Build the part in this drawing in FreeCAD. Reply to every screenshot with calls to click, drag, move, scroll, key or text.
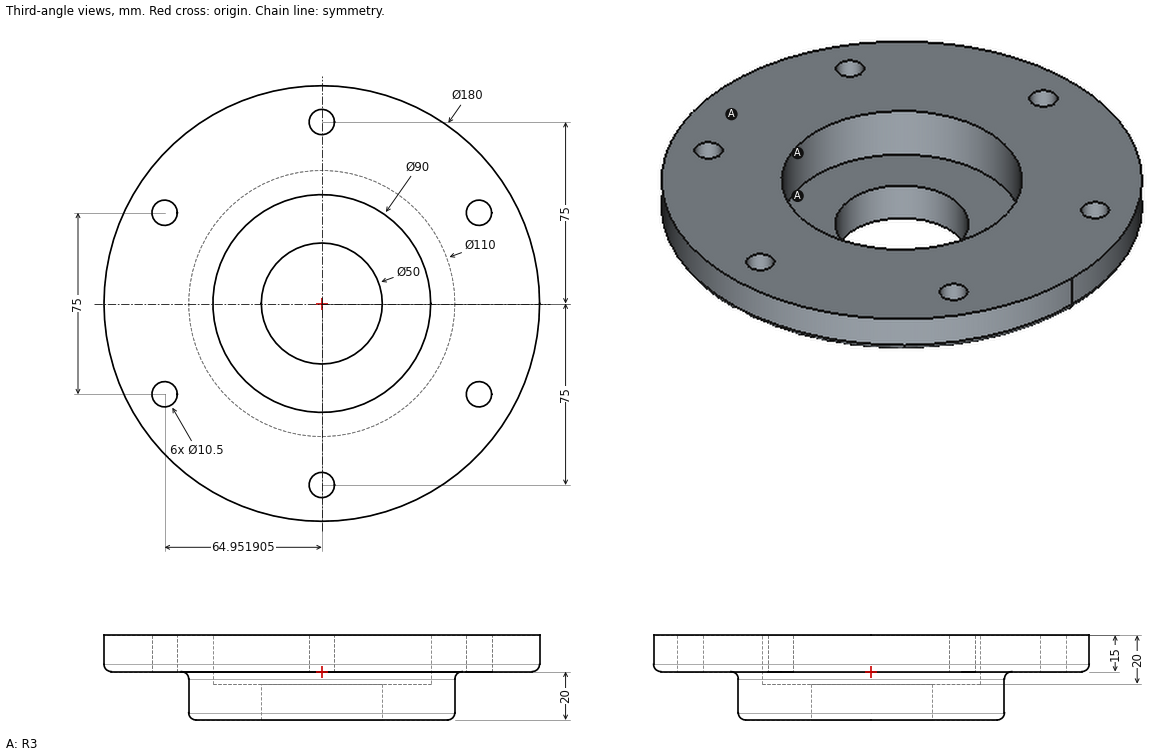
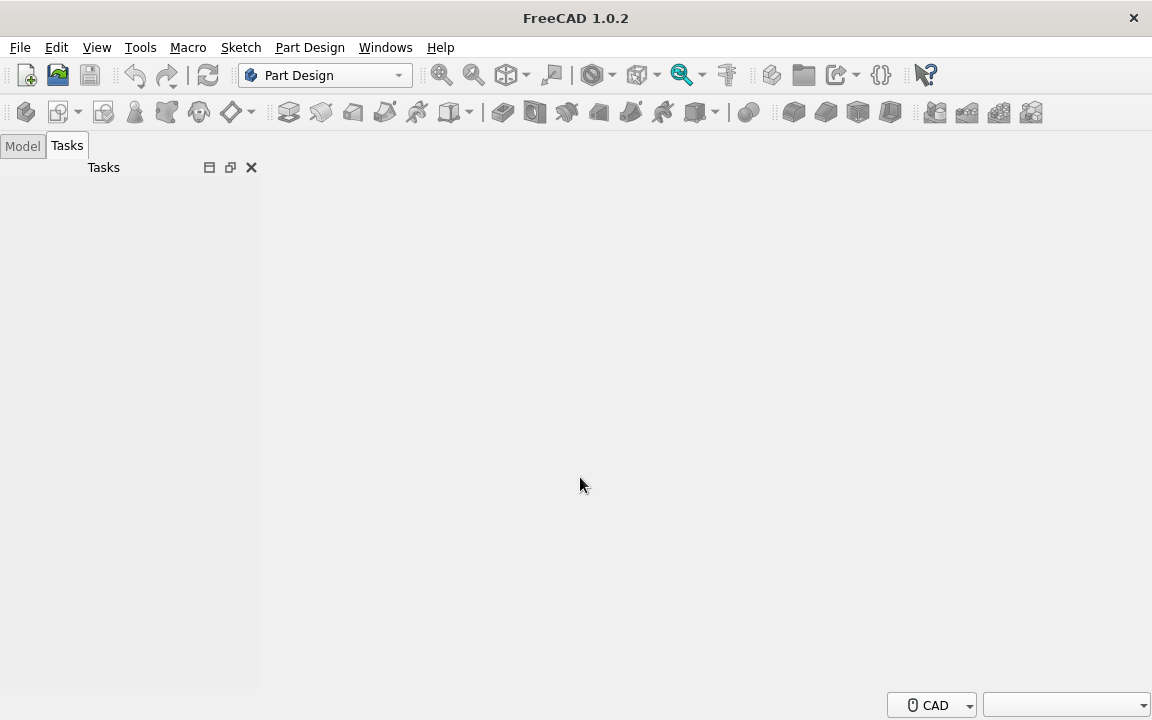
key(ctrl+n)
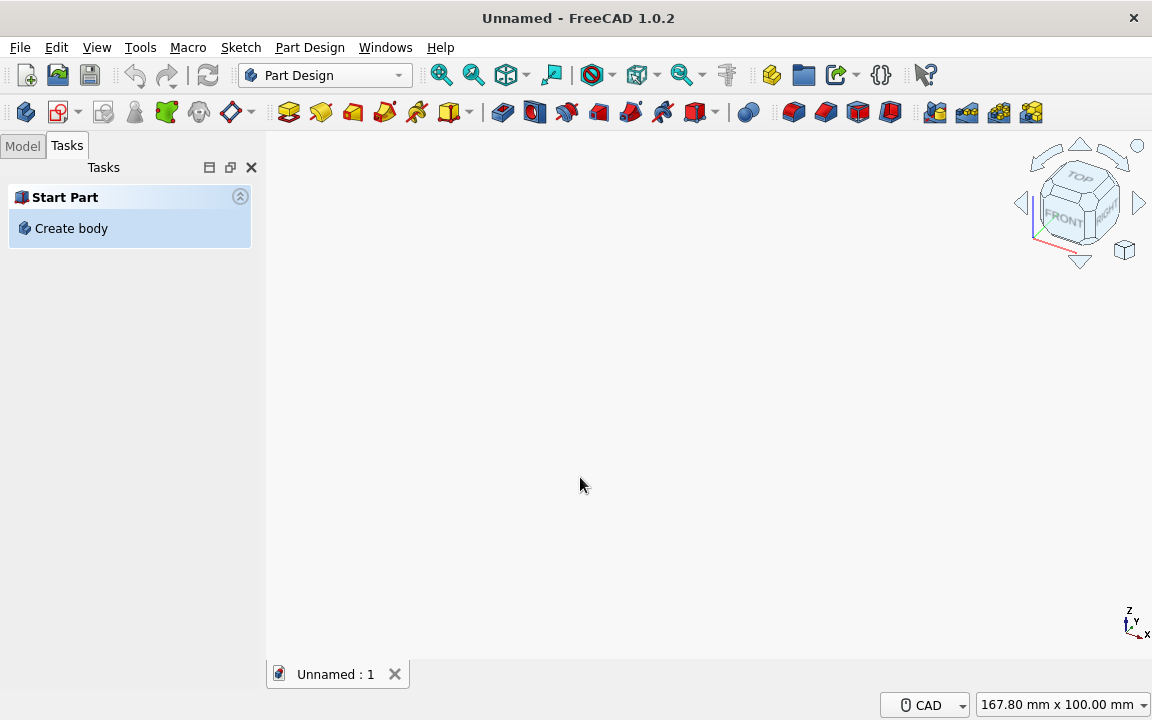
click(58, 112)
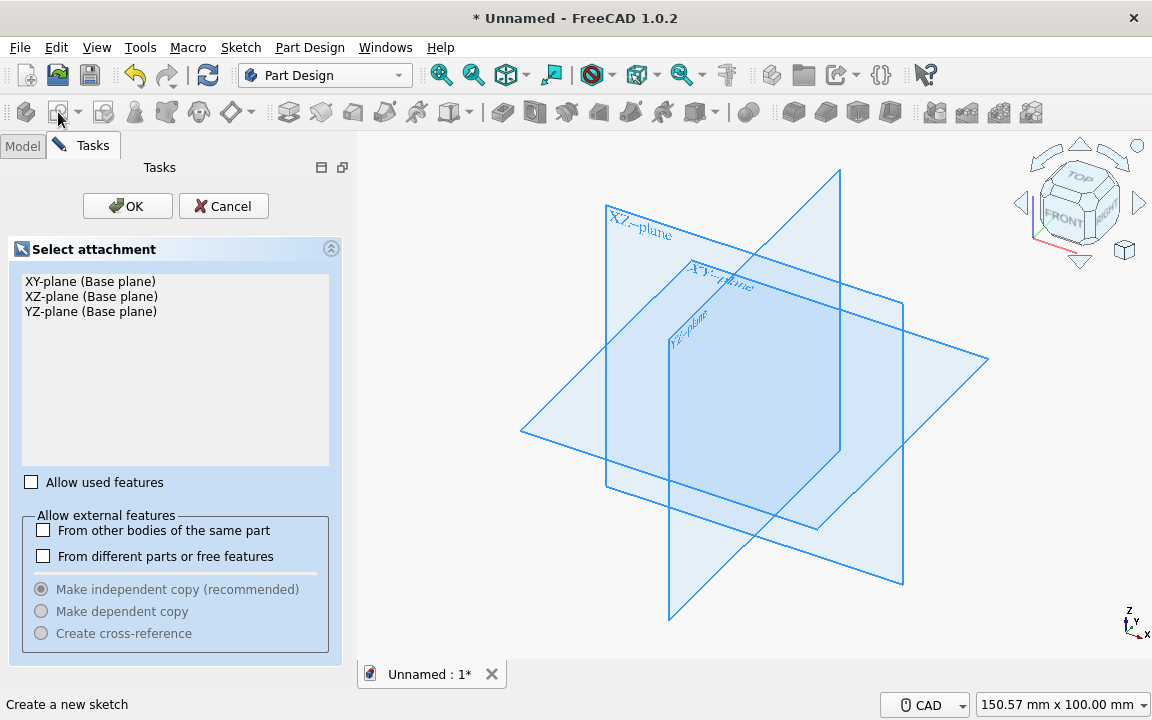
click(82, 282)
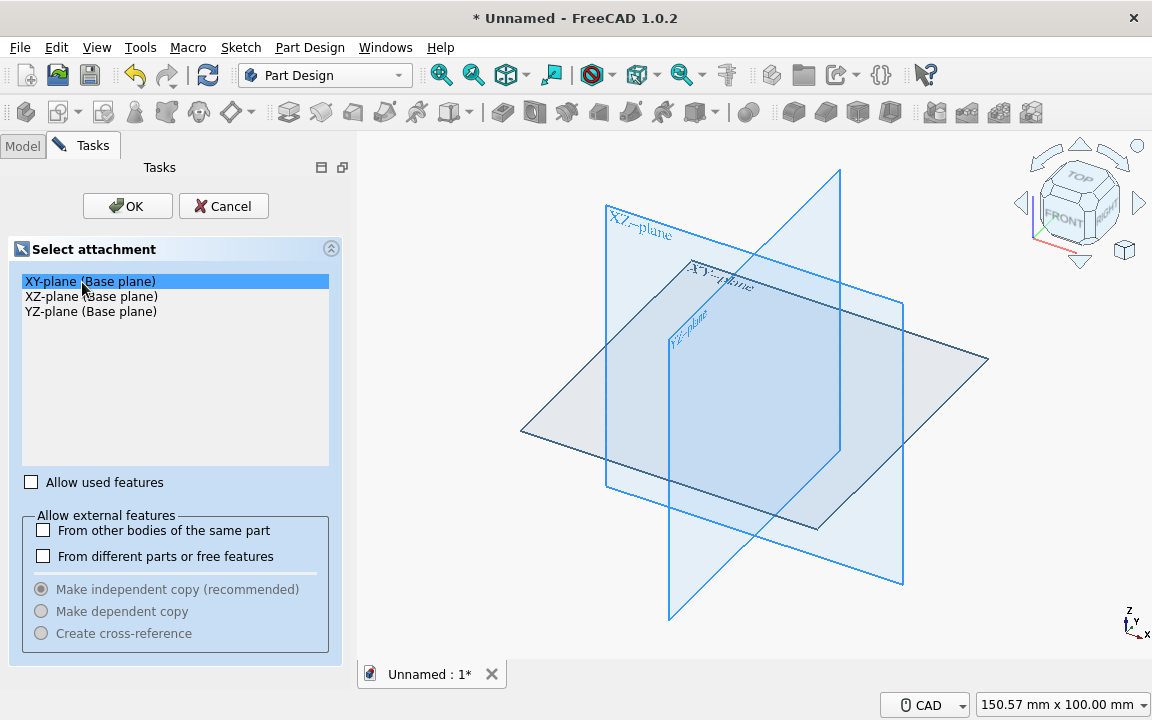
click(128, 206)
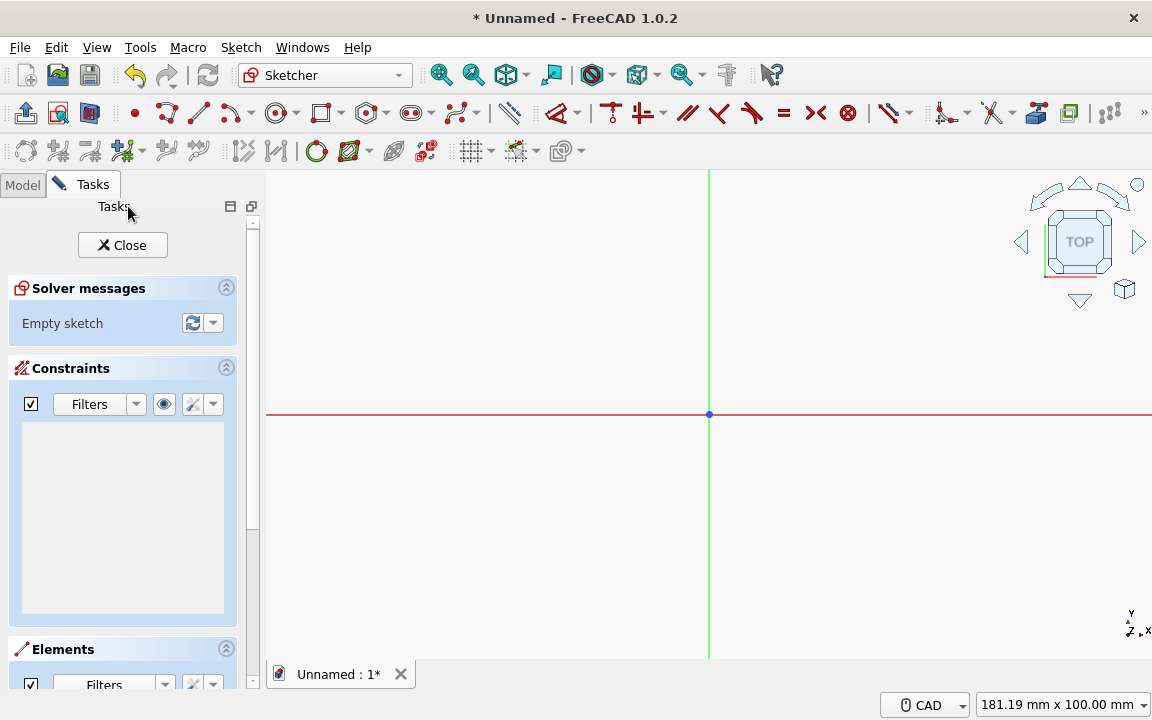
scroll(601, 414, down, 5)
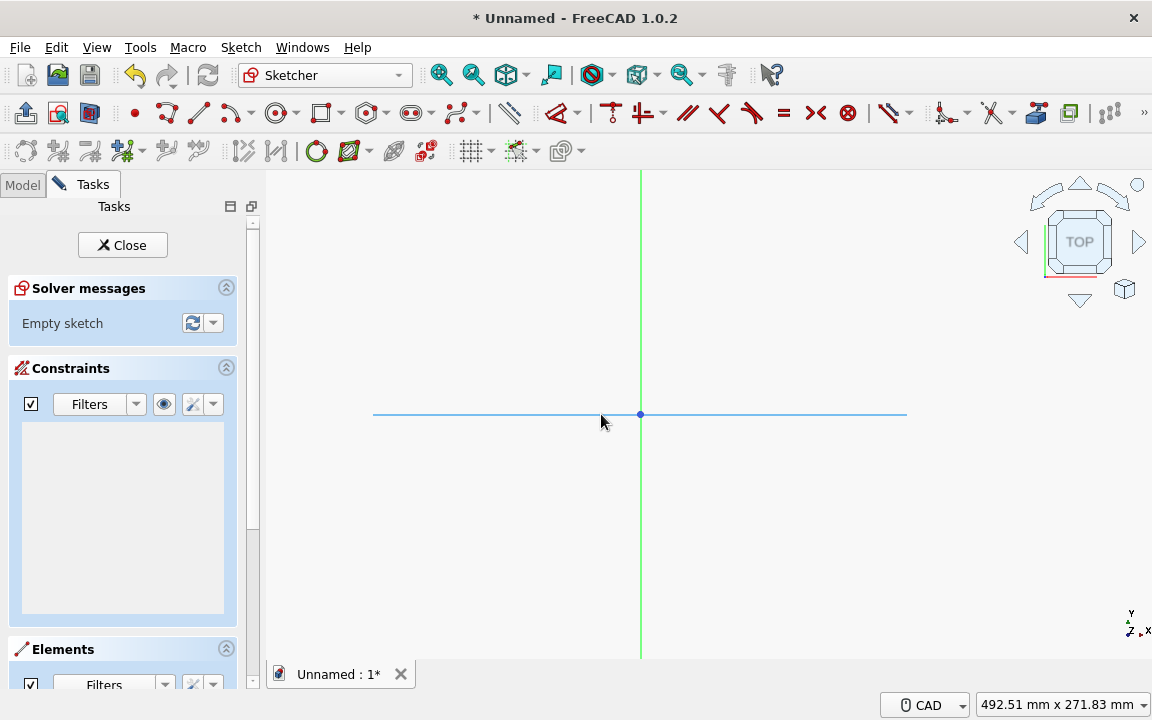
key(g)
key(c)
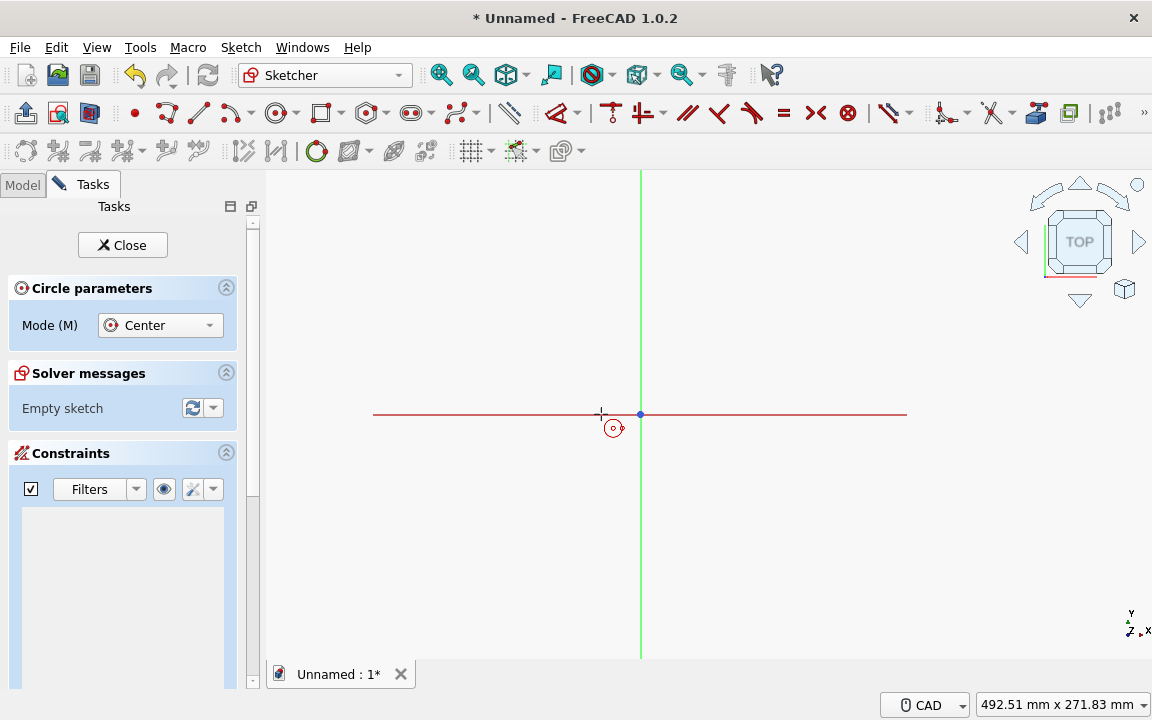
click(641, 414)
move(755, 300)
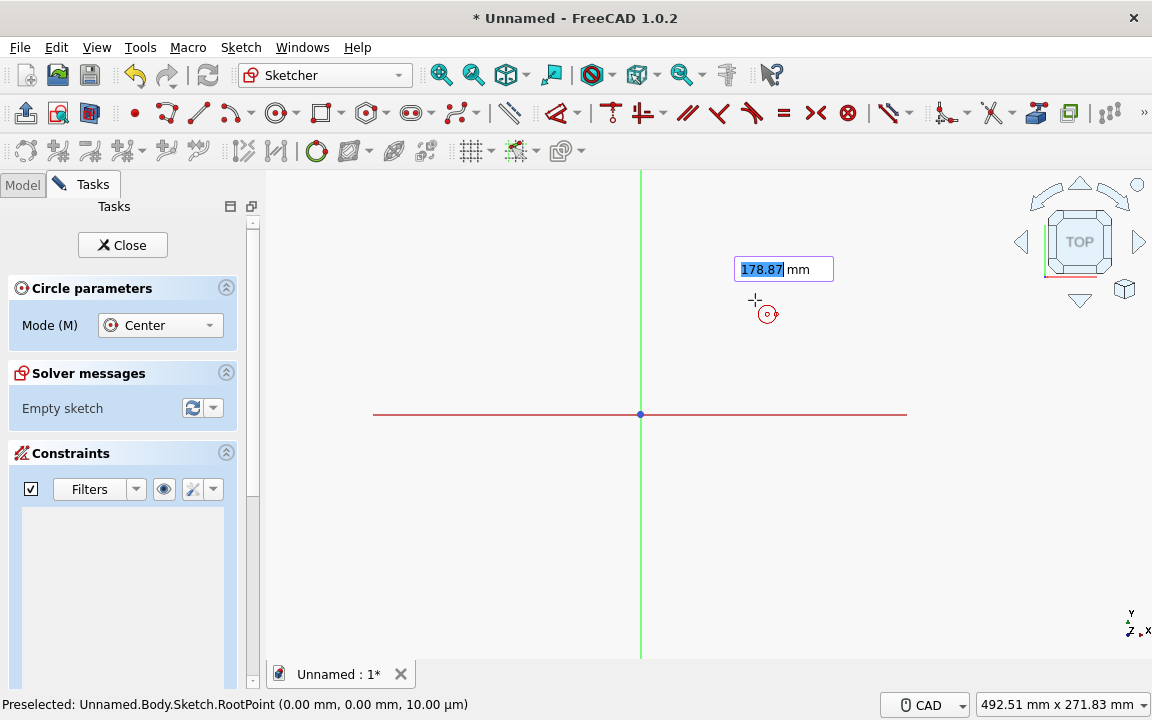
text(180)
key(Return)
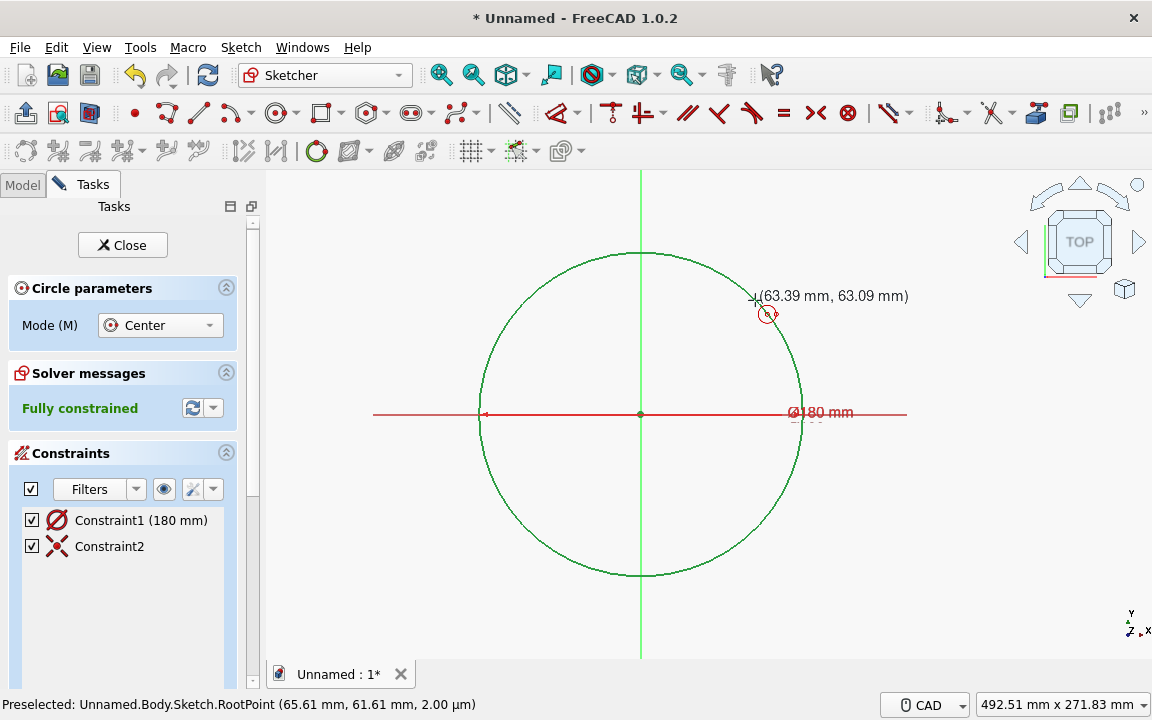
scroll(524, 482, up, 5)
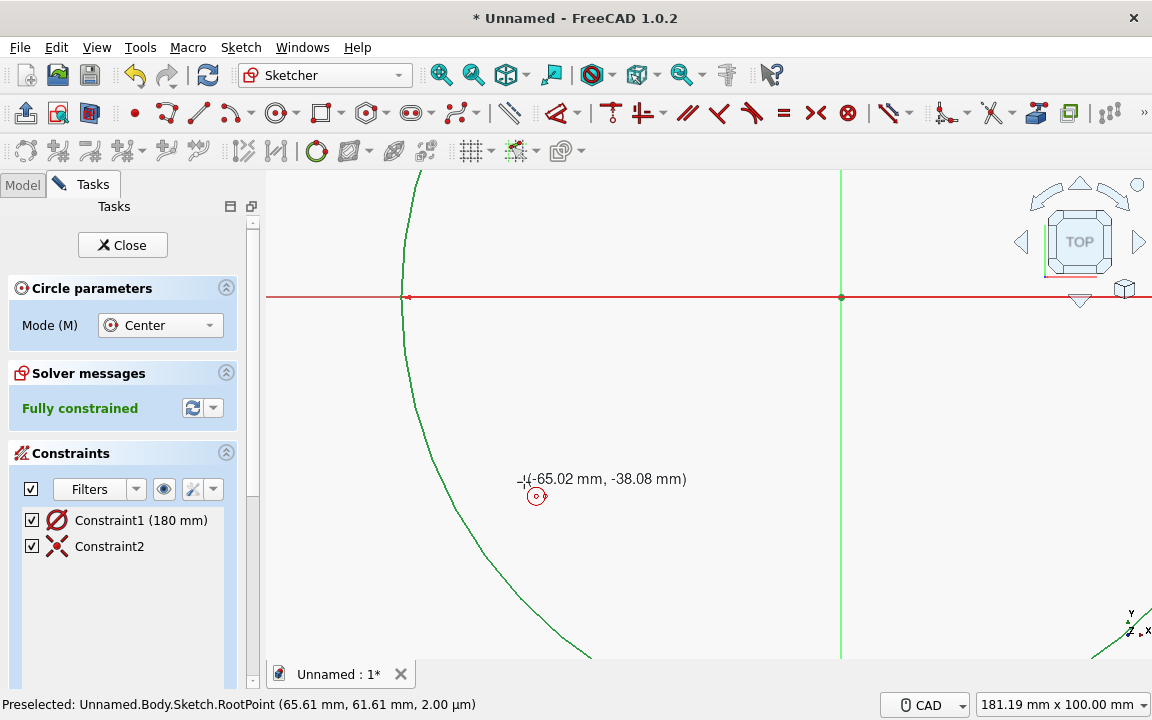
click(524, 481)
move(542, 463)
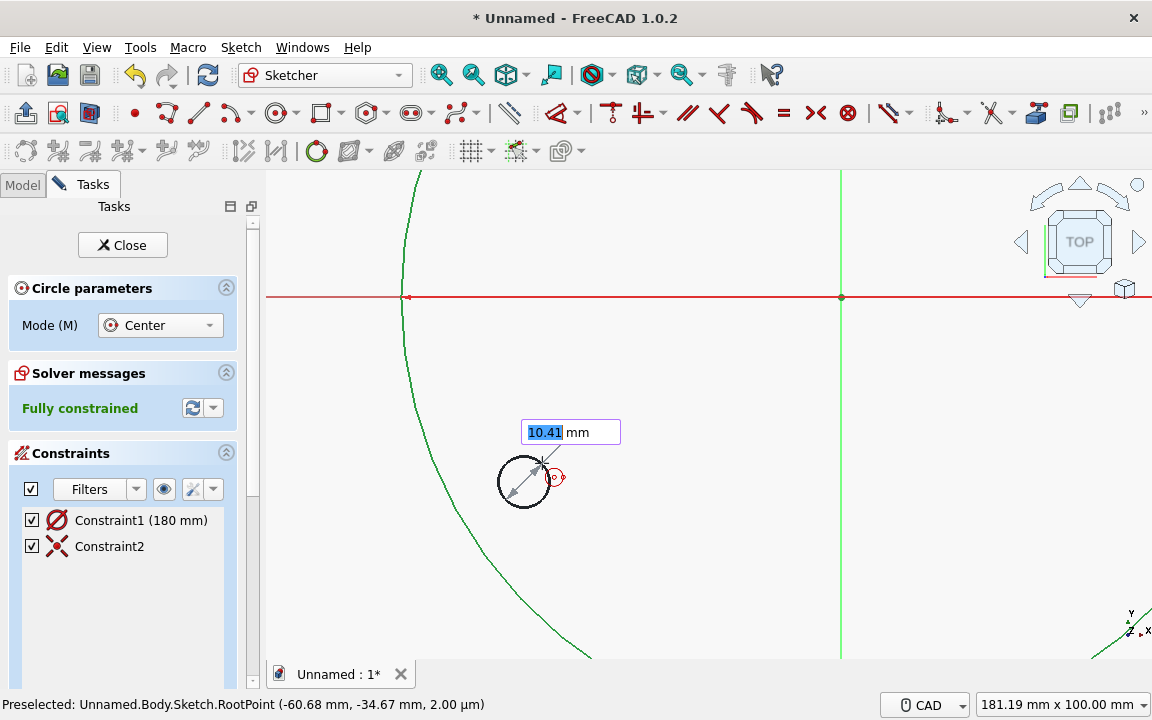
text(10.5)
key(Return)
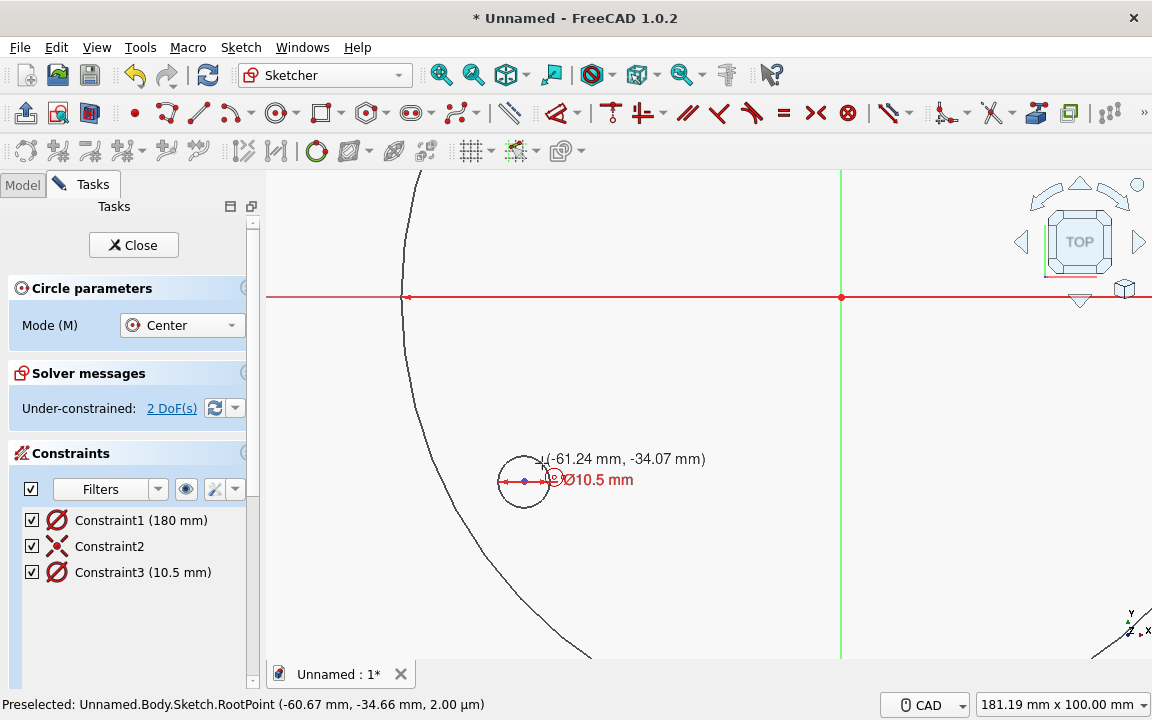
scroll(524, 483, down, 5)